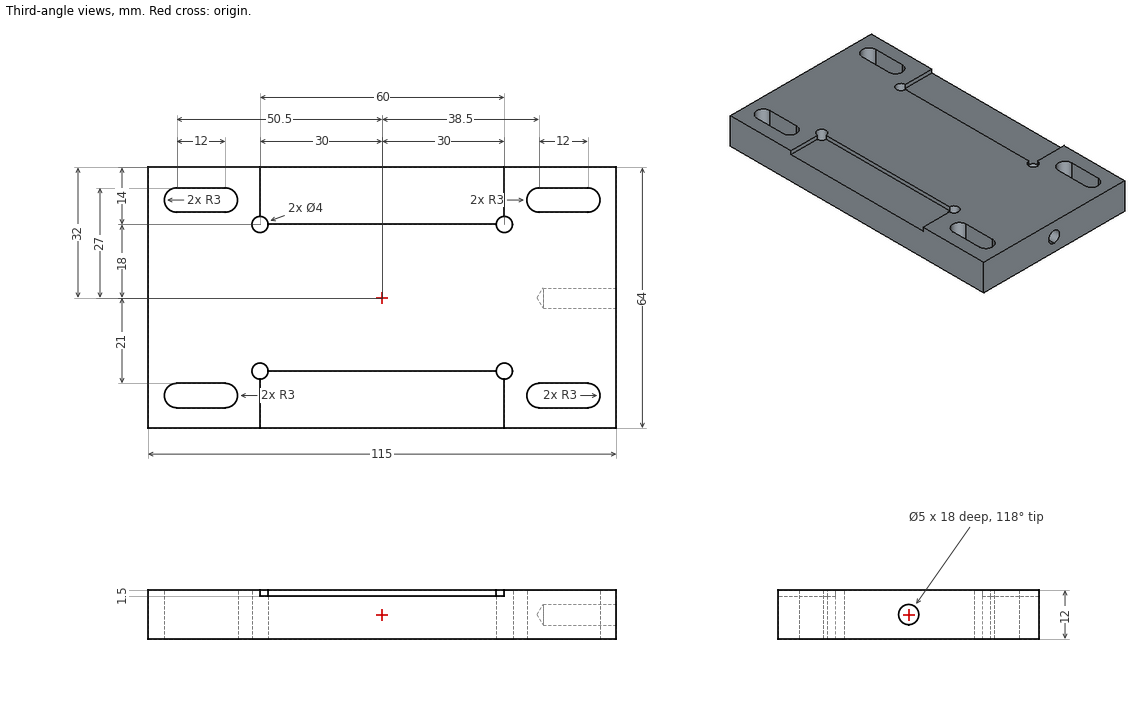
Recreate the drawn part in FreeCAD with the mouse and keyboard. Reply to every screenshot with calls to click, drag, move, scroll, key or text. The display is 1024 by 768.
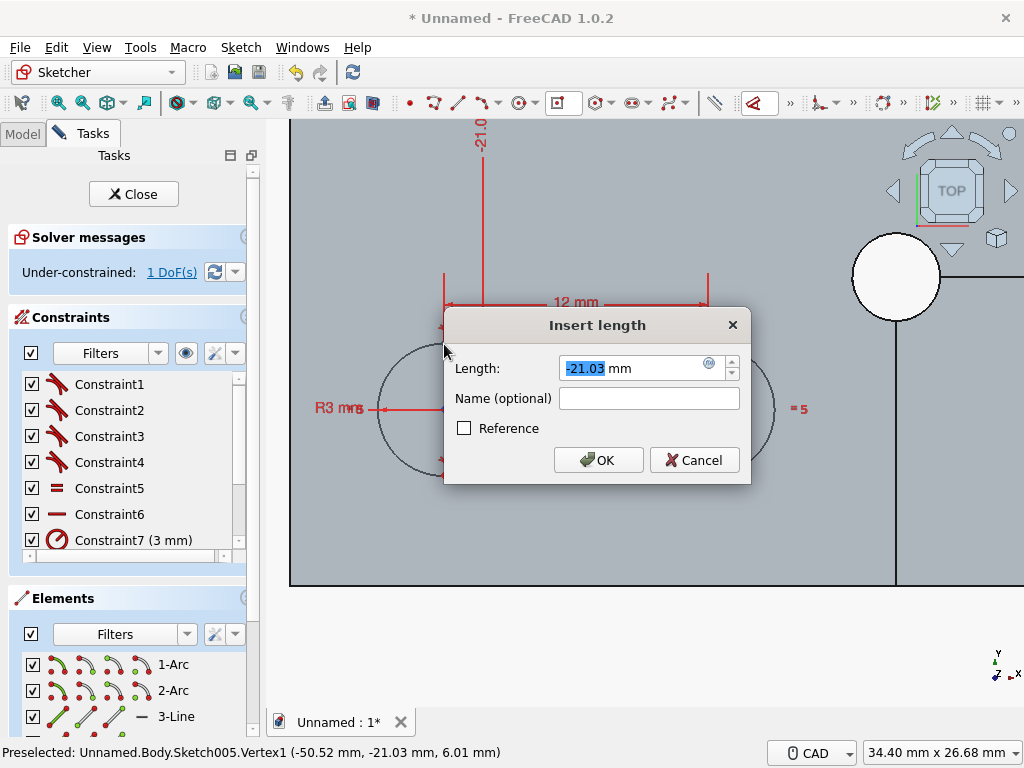
text(-21)
key(Return)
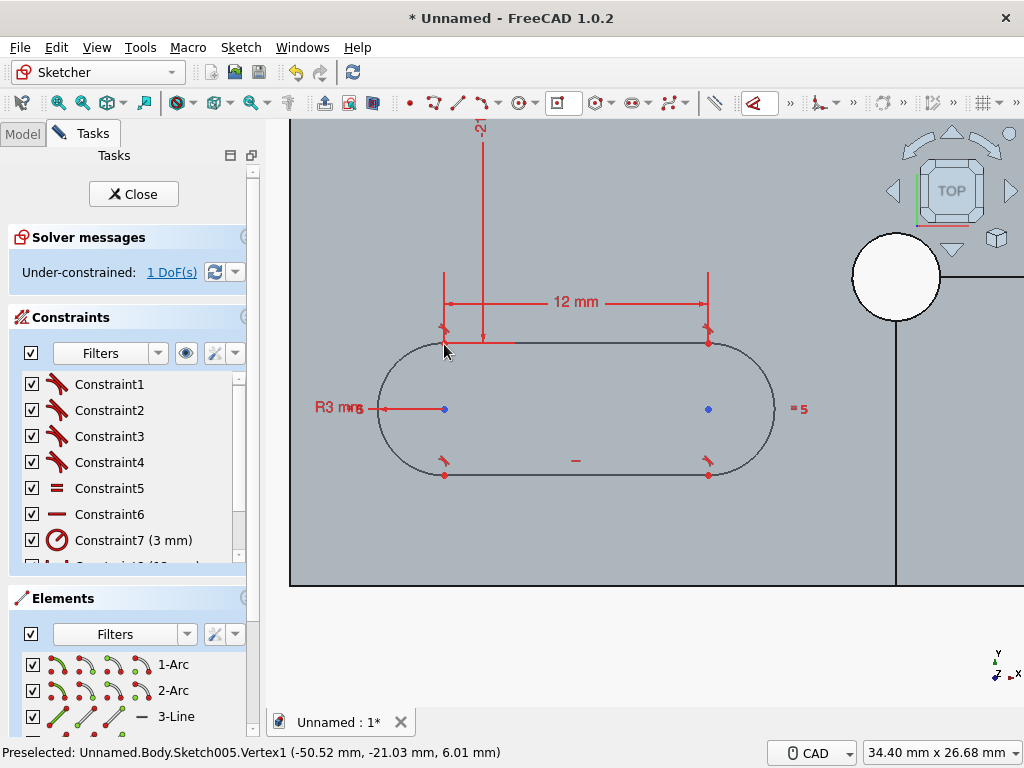
click(444, 343)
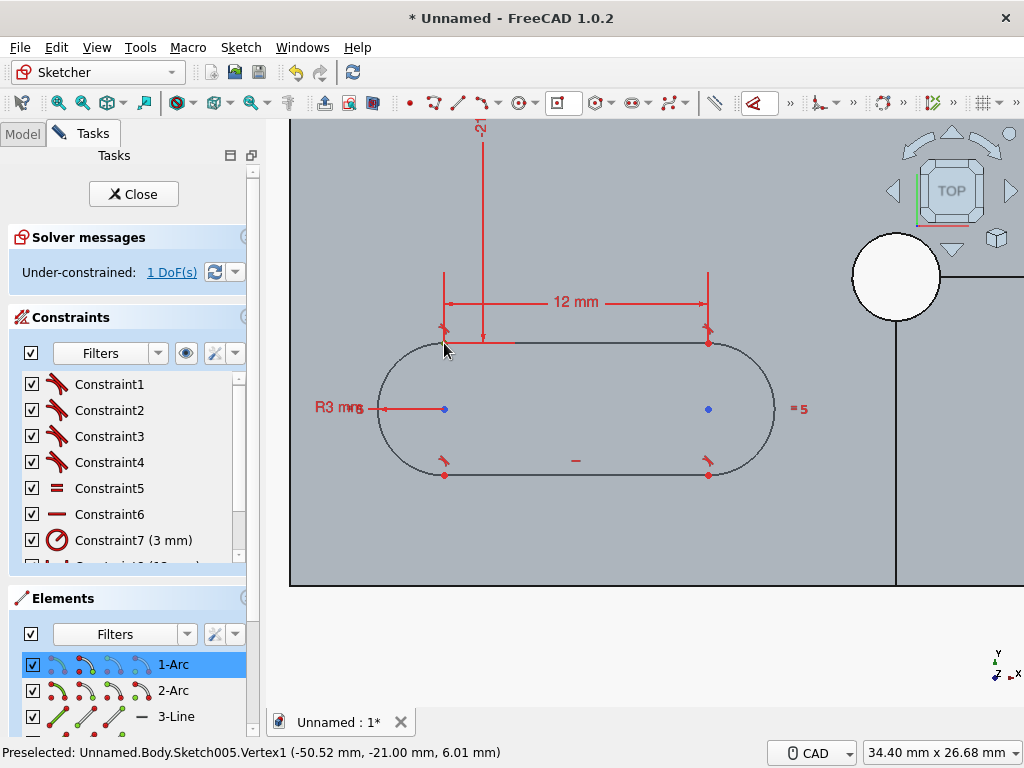
click(772, 104)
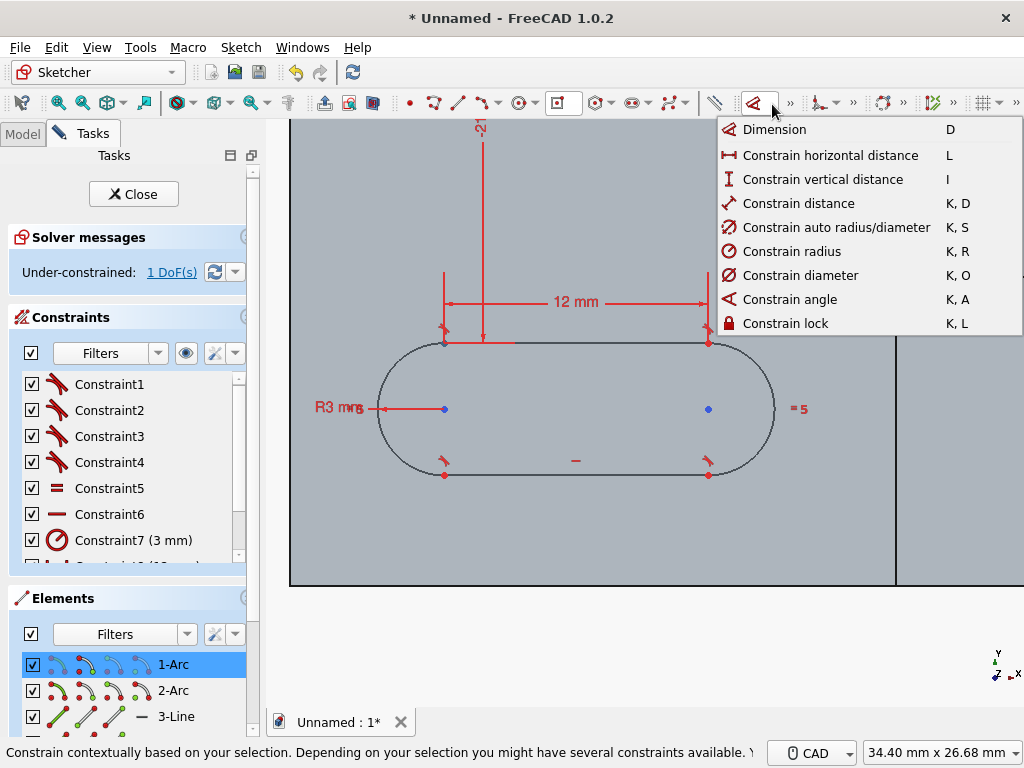
click(870, 155)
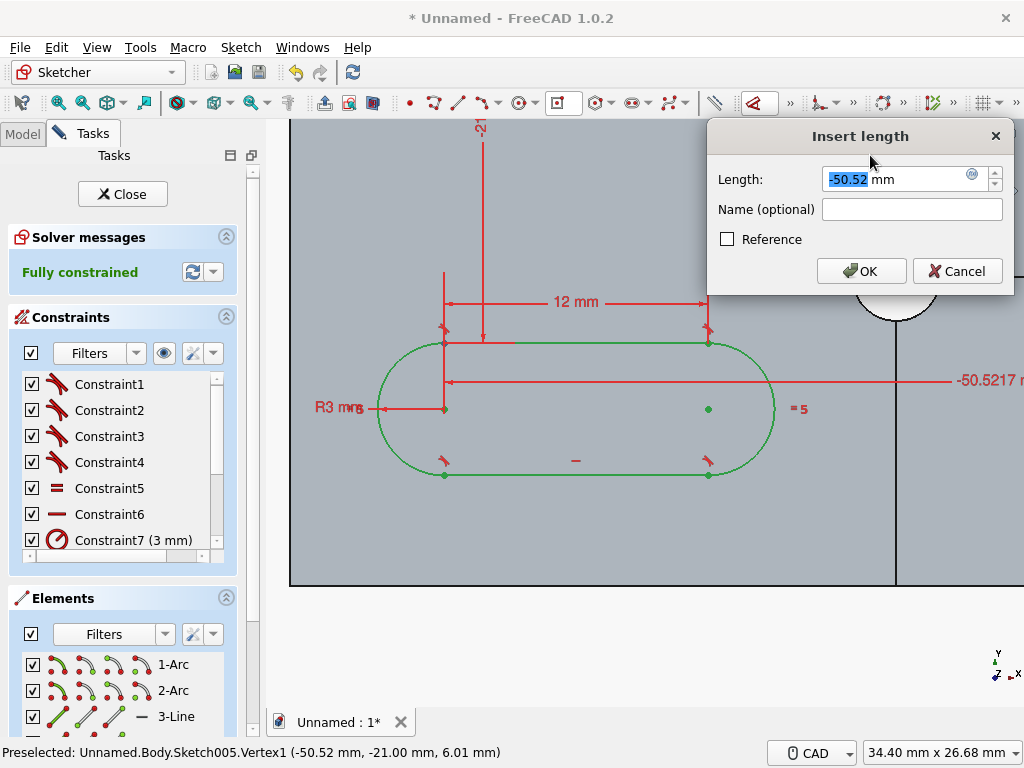
text(-50.5)
key(Return)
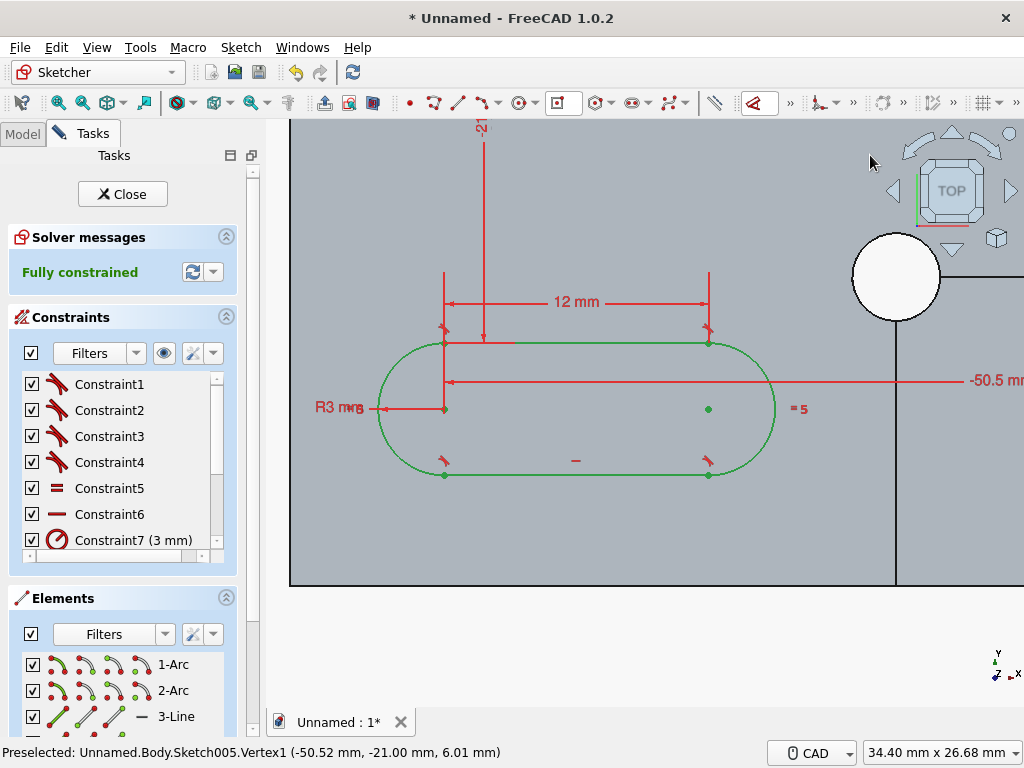
click(123, 194)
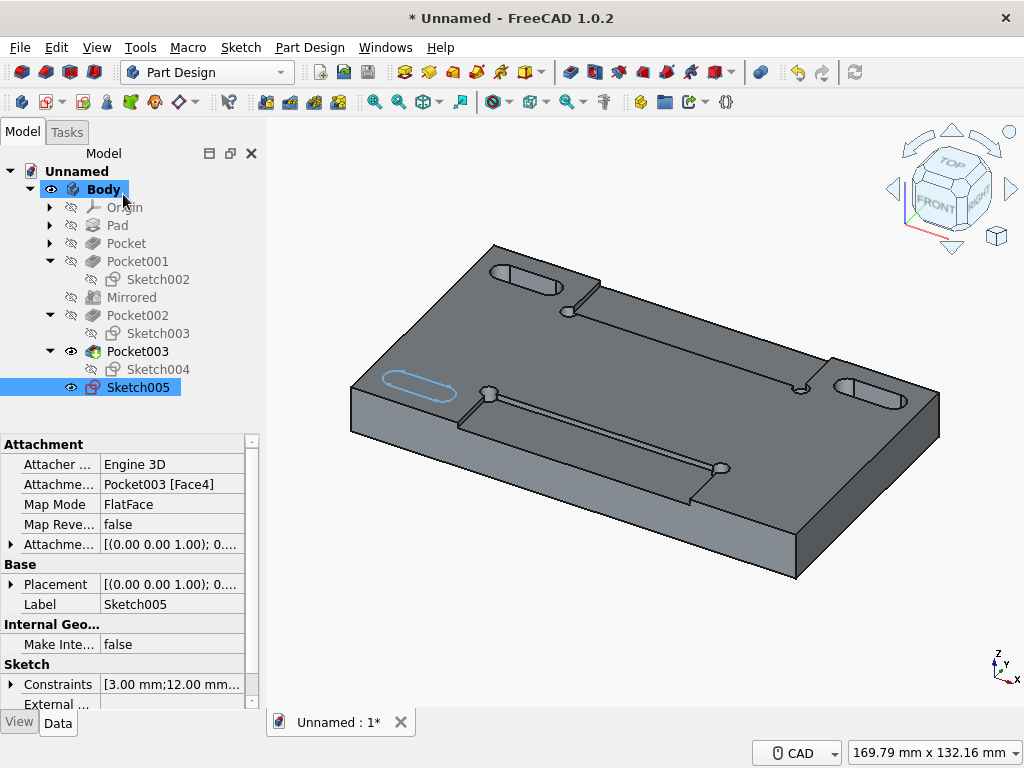
click(572, 72)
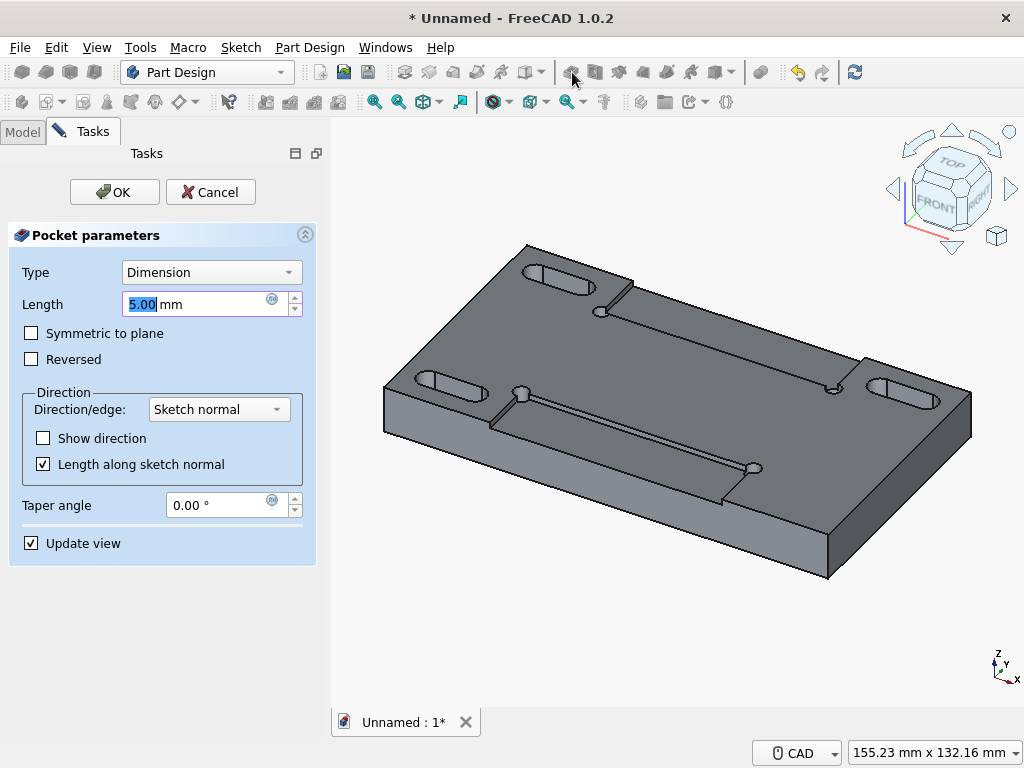
click(212, 272)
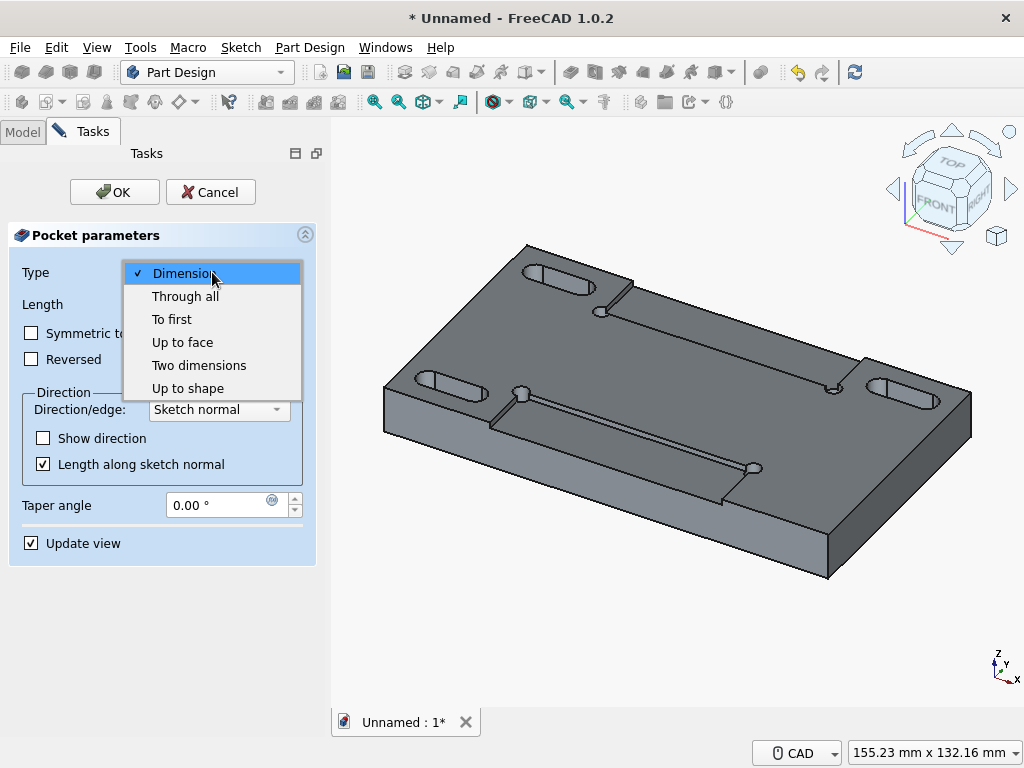
click(212, 320)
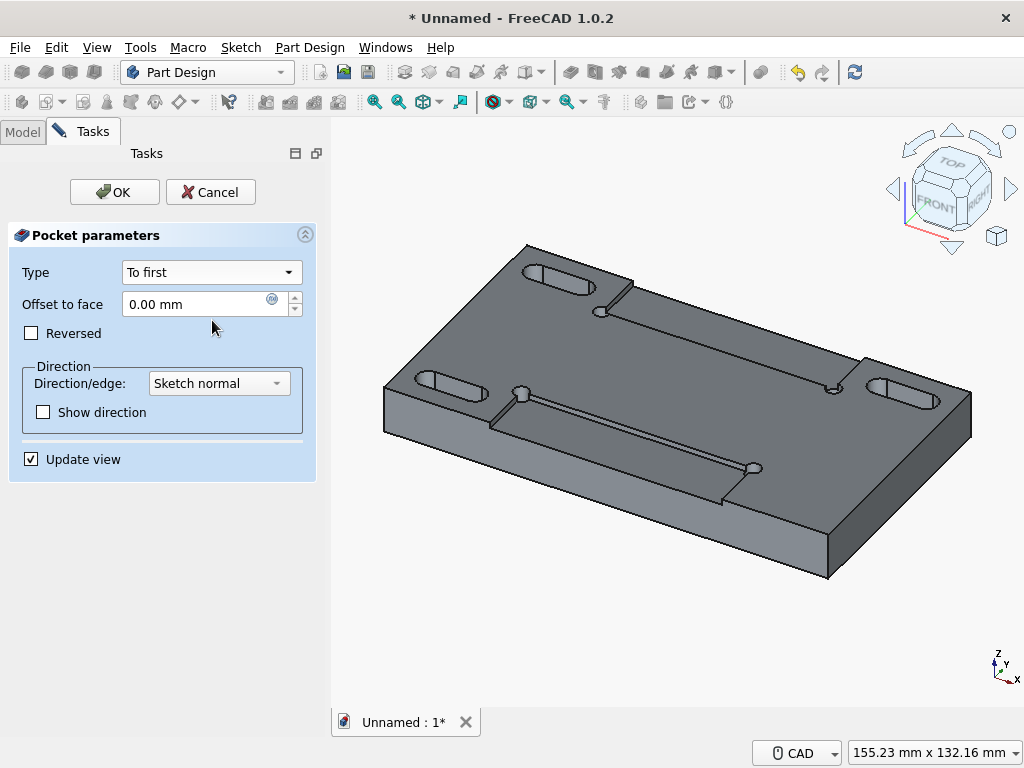
click(115, 192)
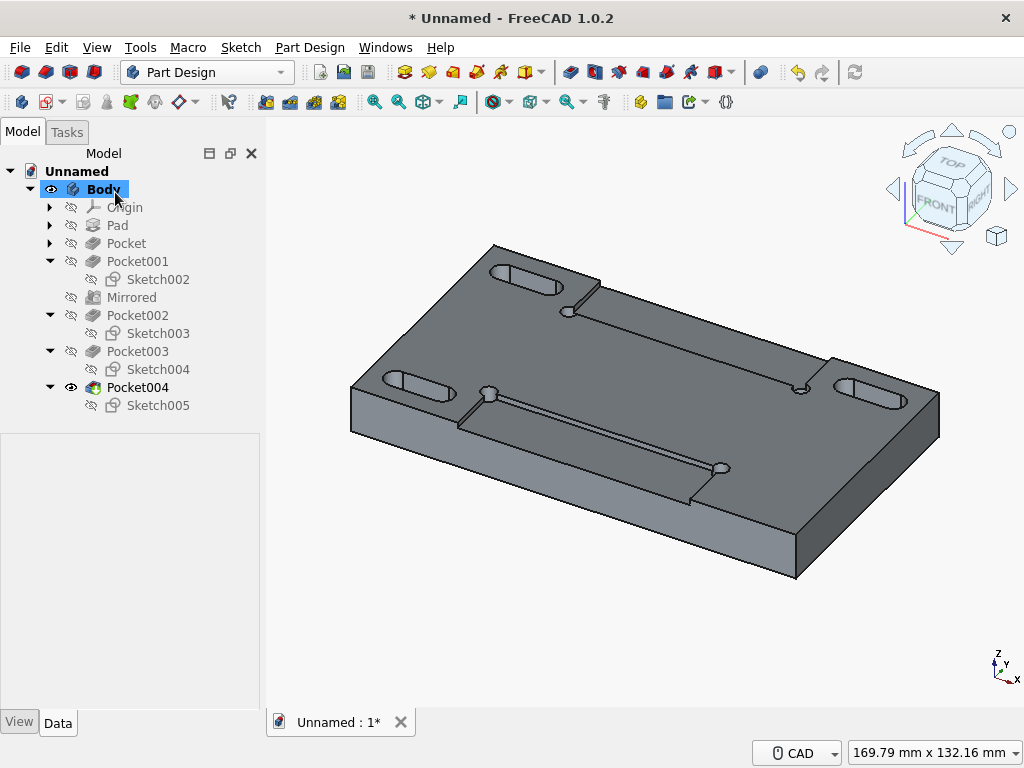
click(709, 410)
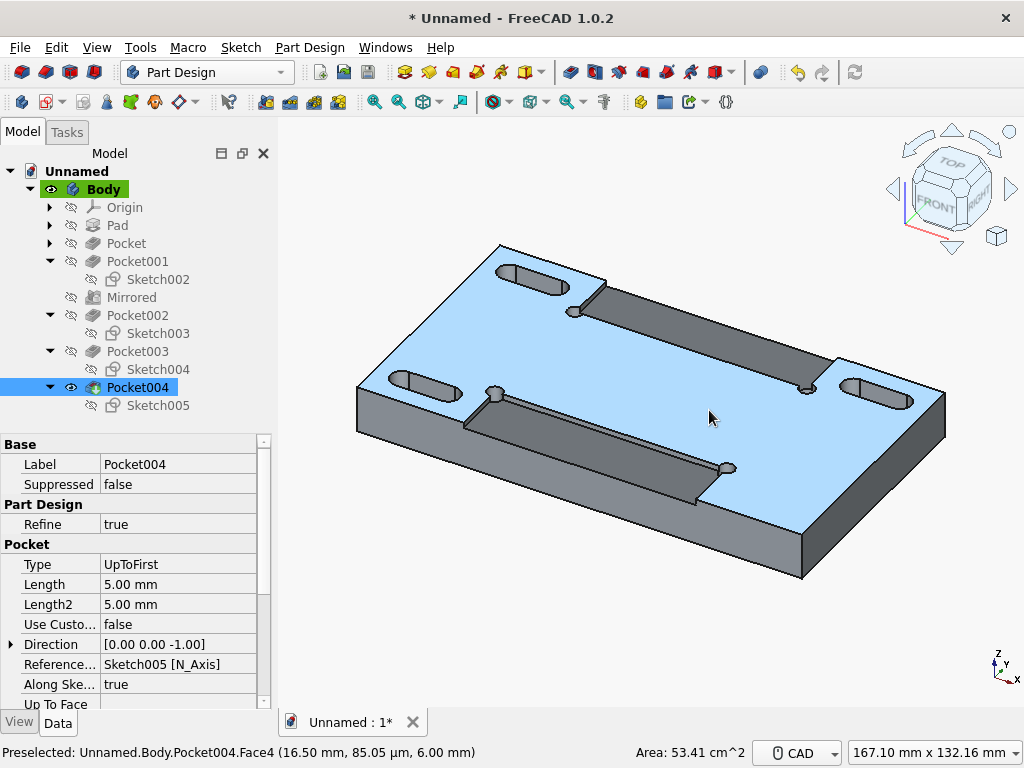
click(46, 102)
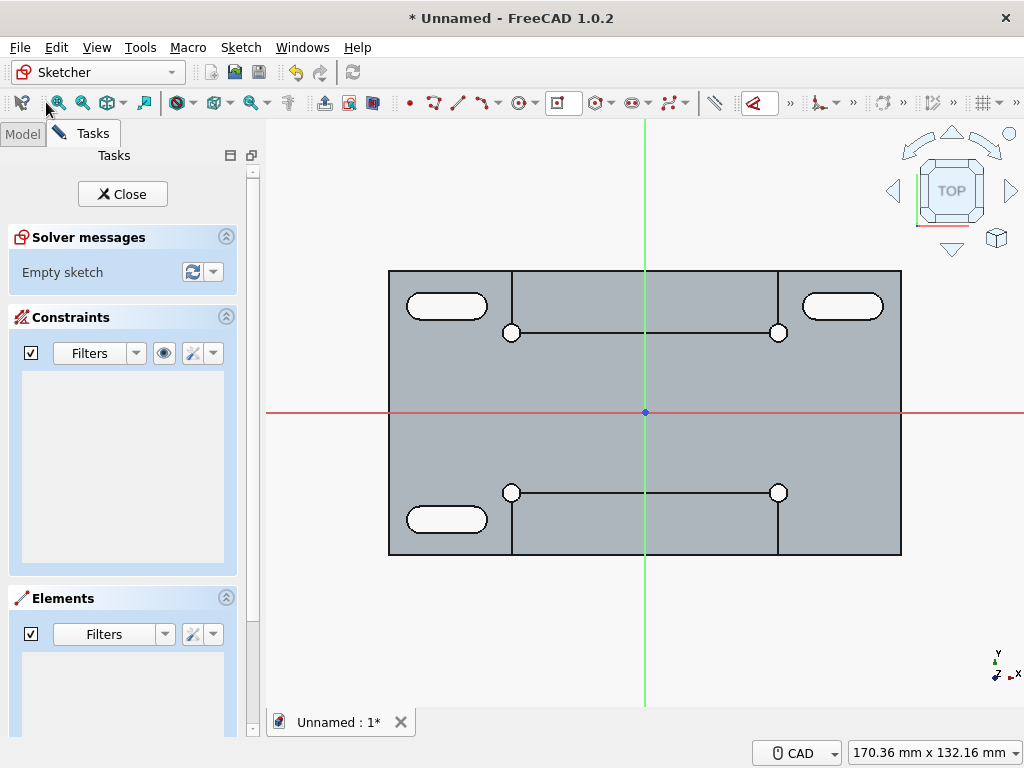
scroll(576, 413, down, 5)